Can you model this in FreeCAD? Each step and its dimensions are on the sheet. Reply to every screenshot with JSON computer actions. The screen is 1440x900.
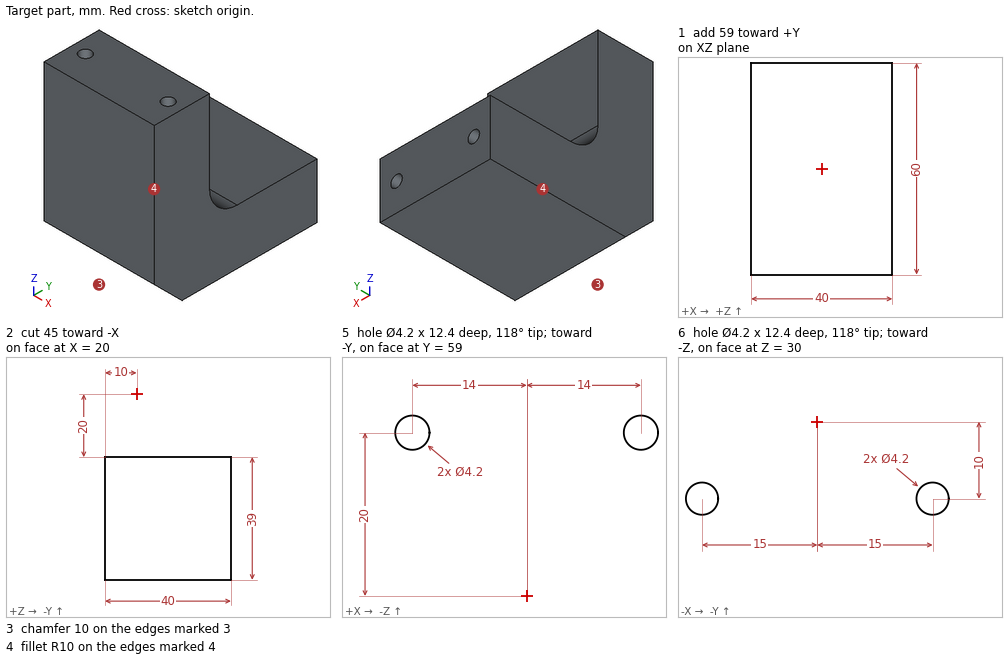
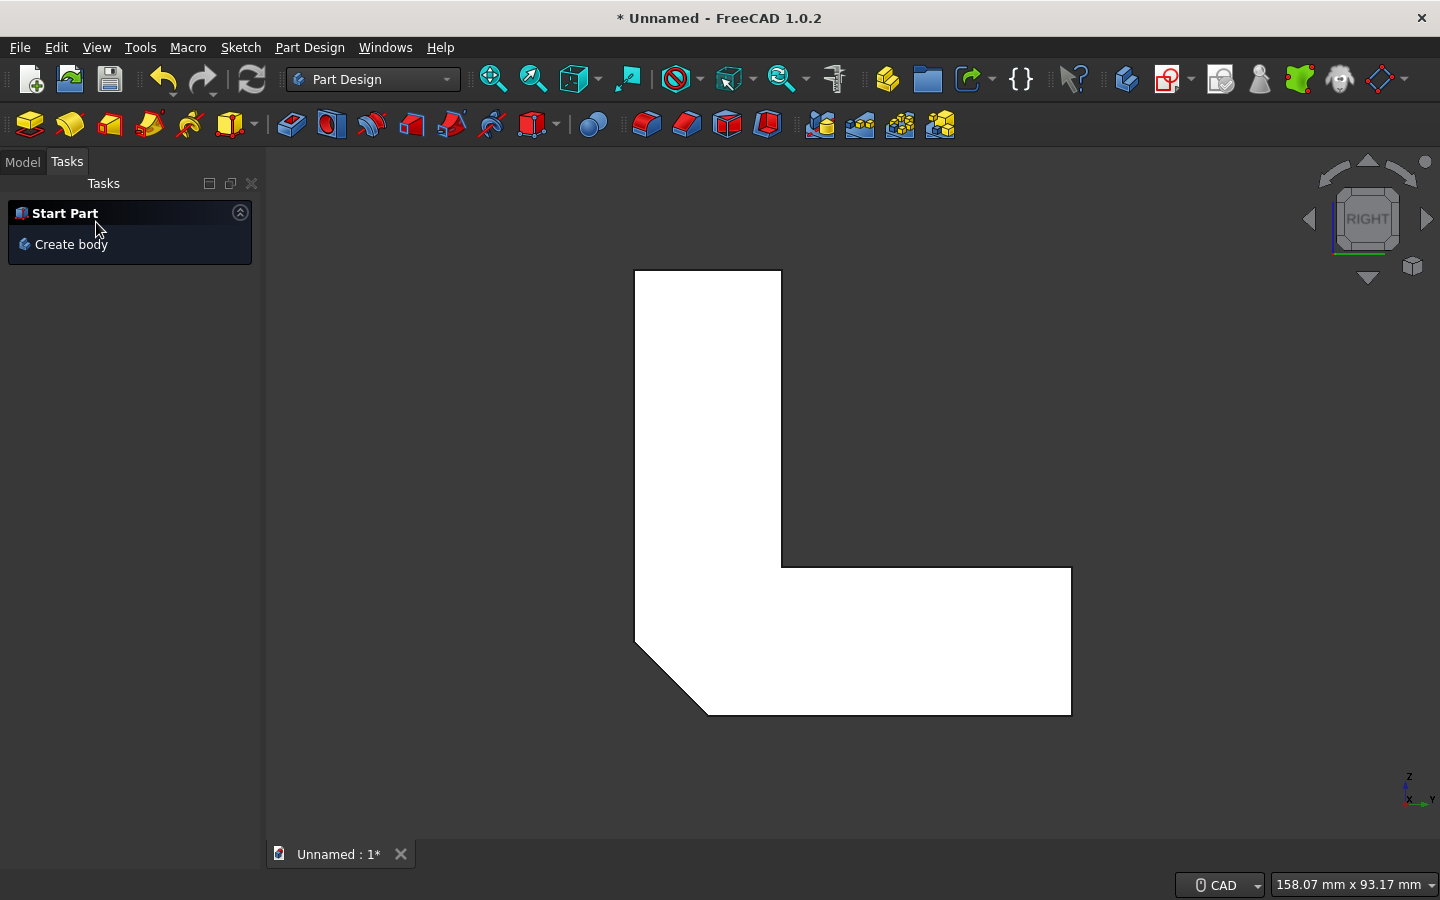
{"action": "key", "text": "5"}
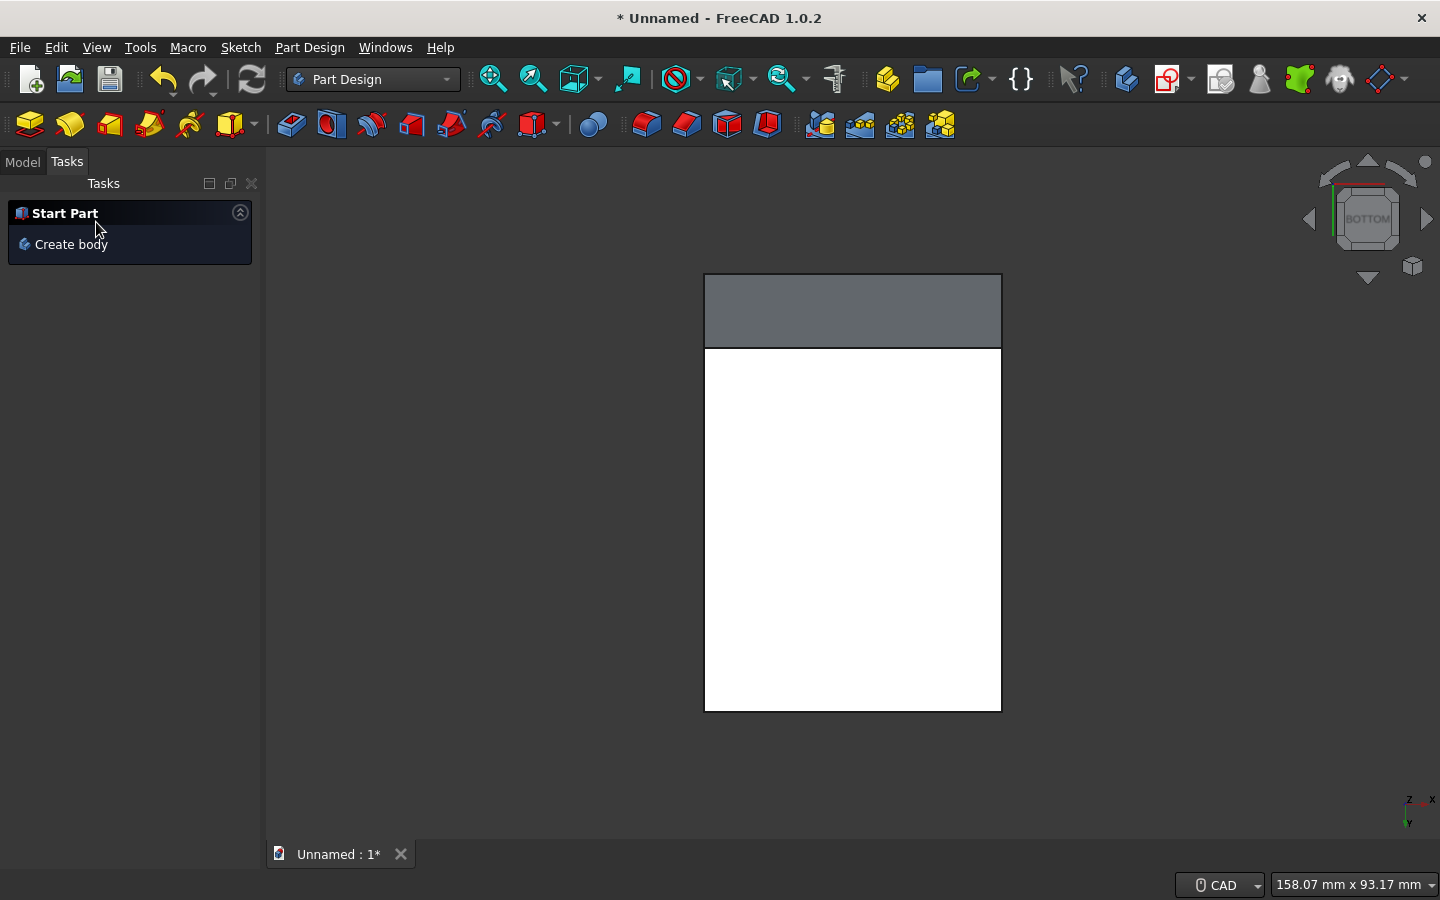
{"action": "key", "text": "4"}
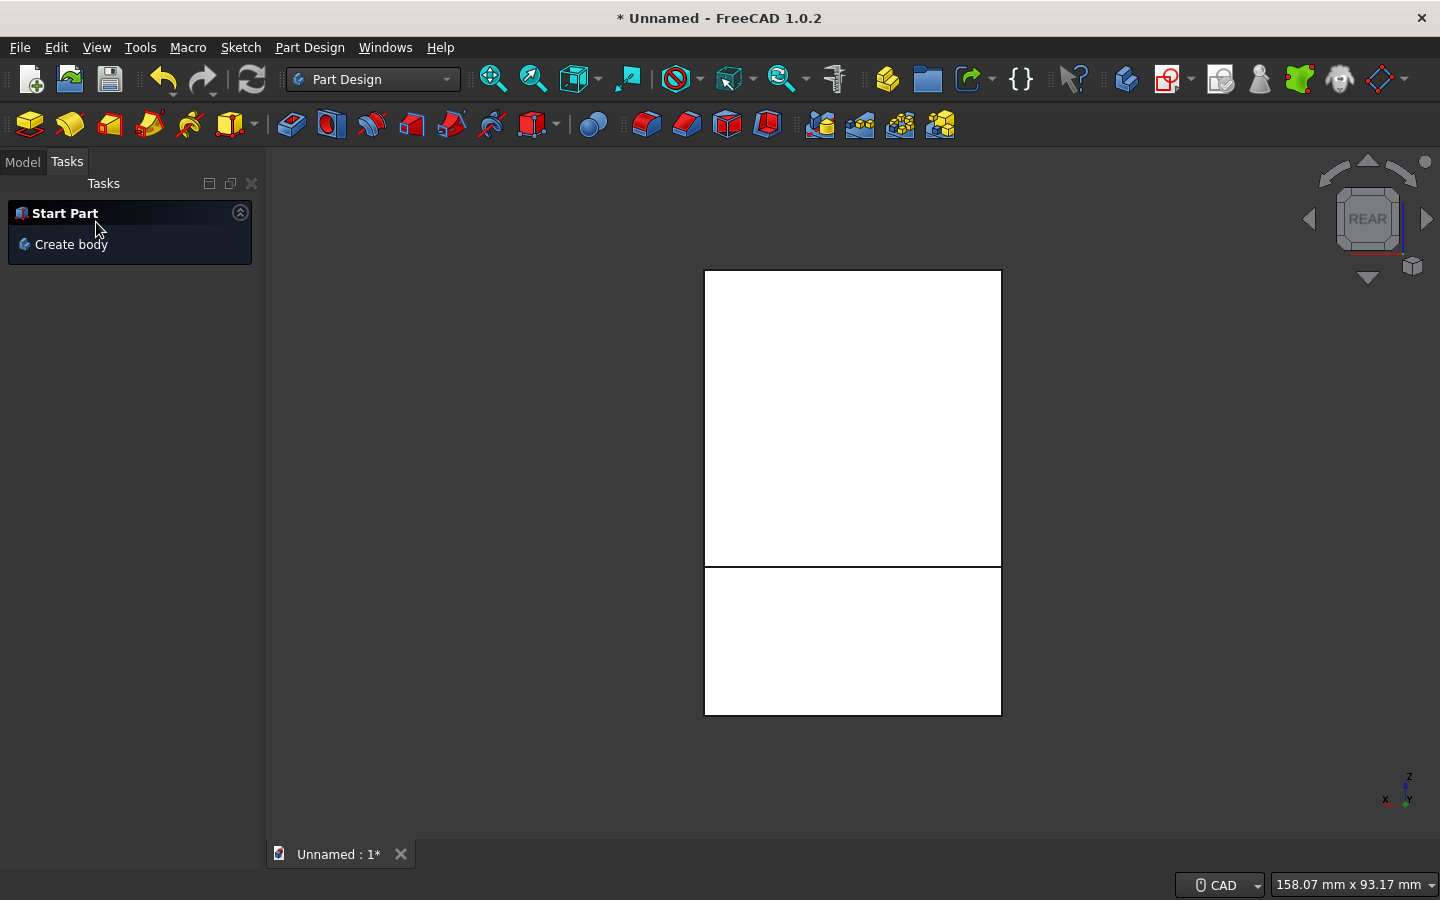
{"action": "key", "text": "6"}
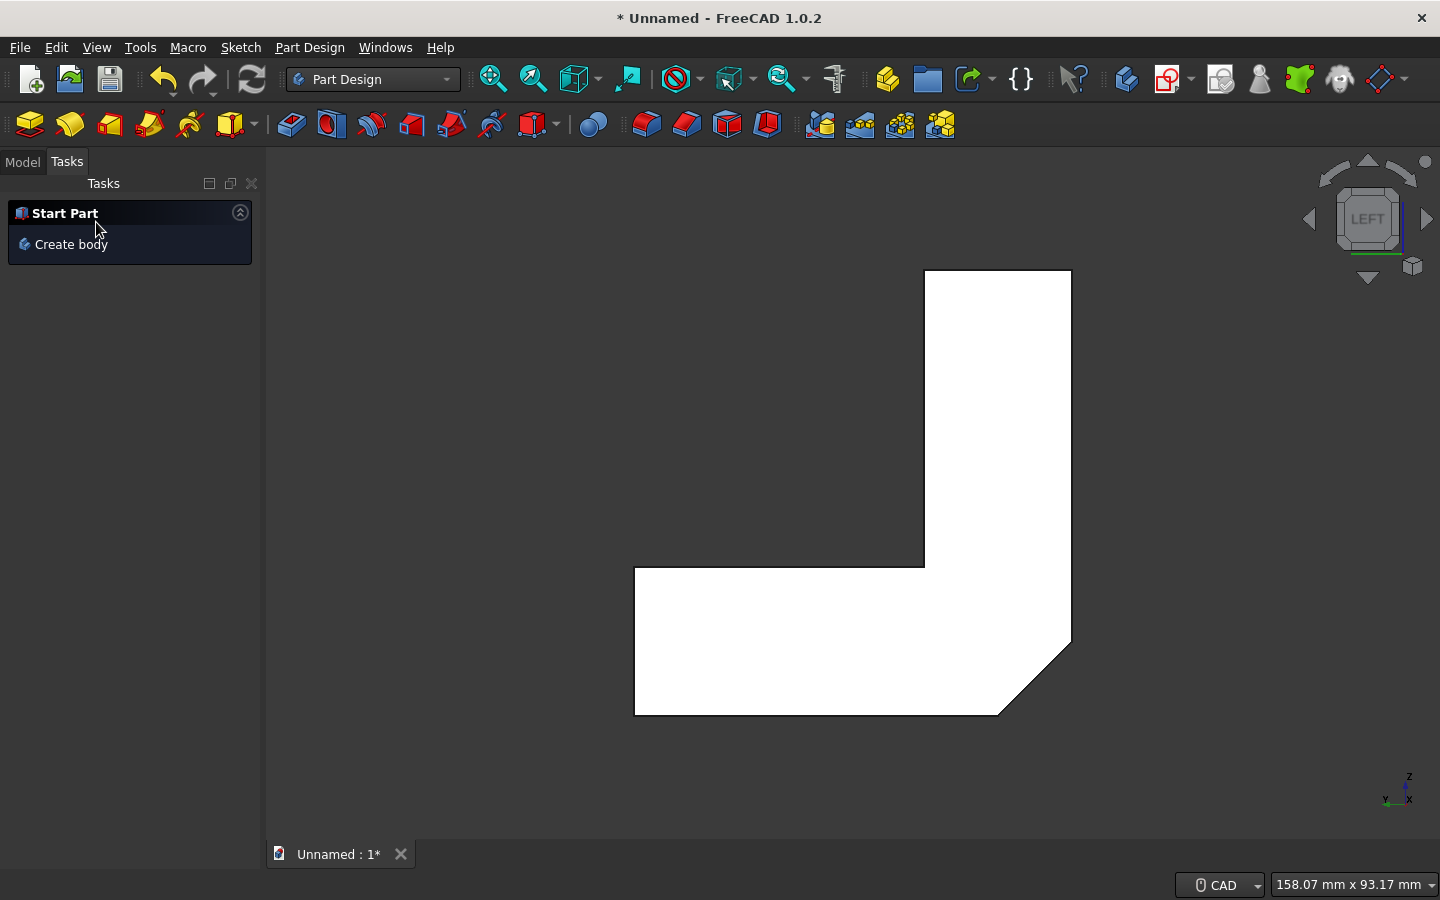
{"action": "key", "text": "v 3"}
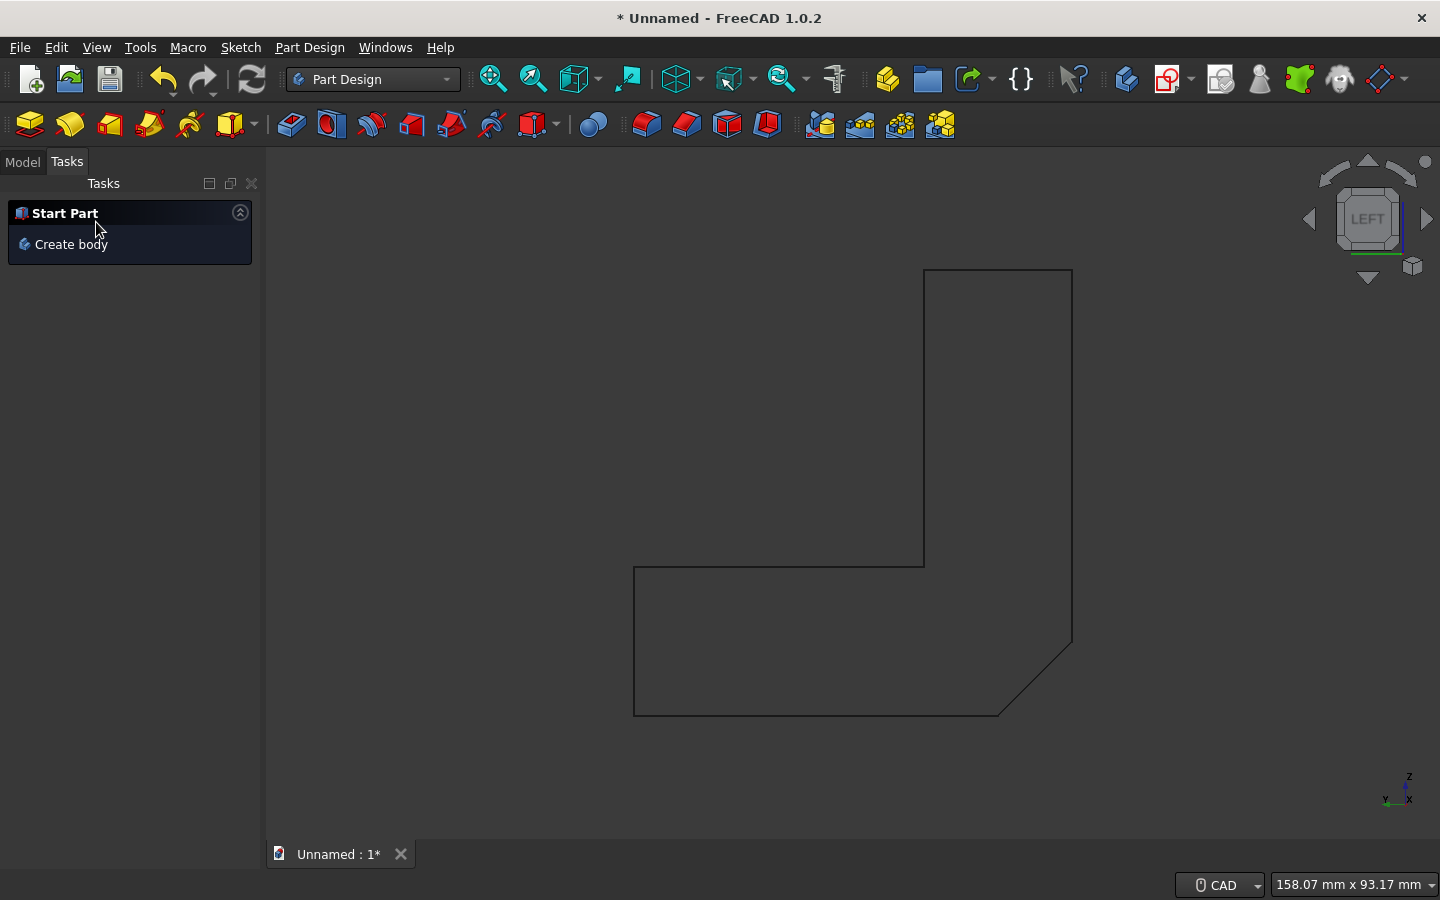
{"action": "key", "text": "0"}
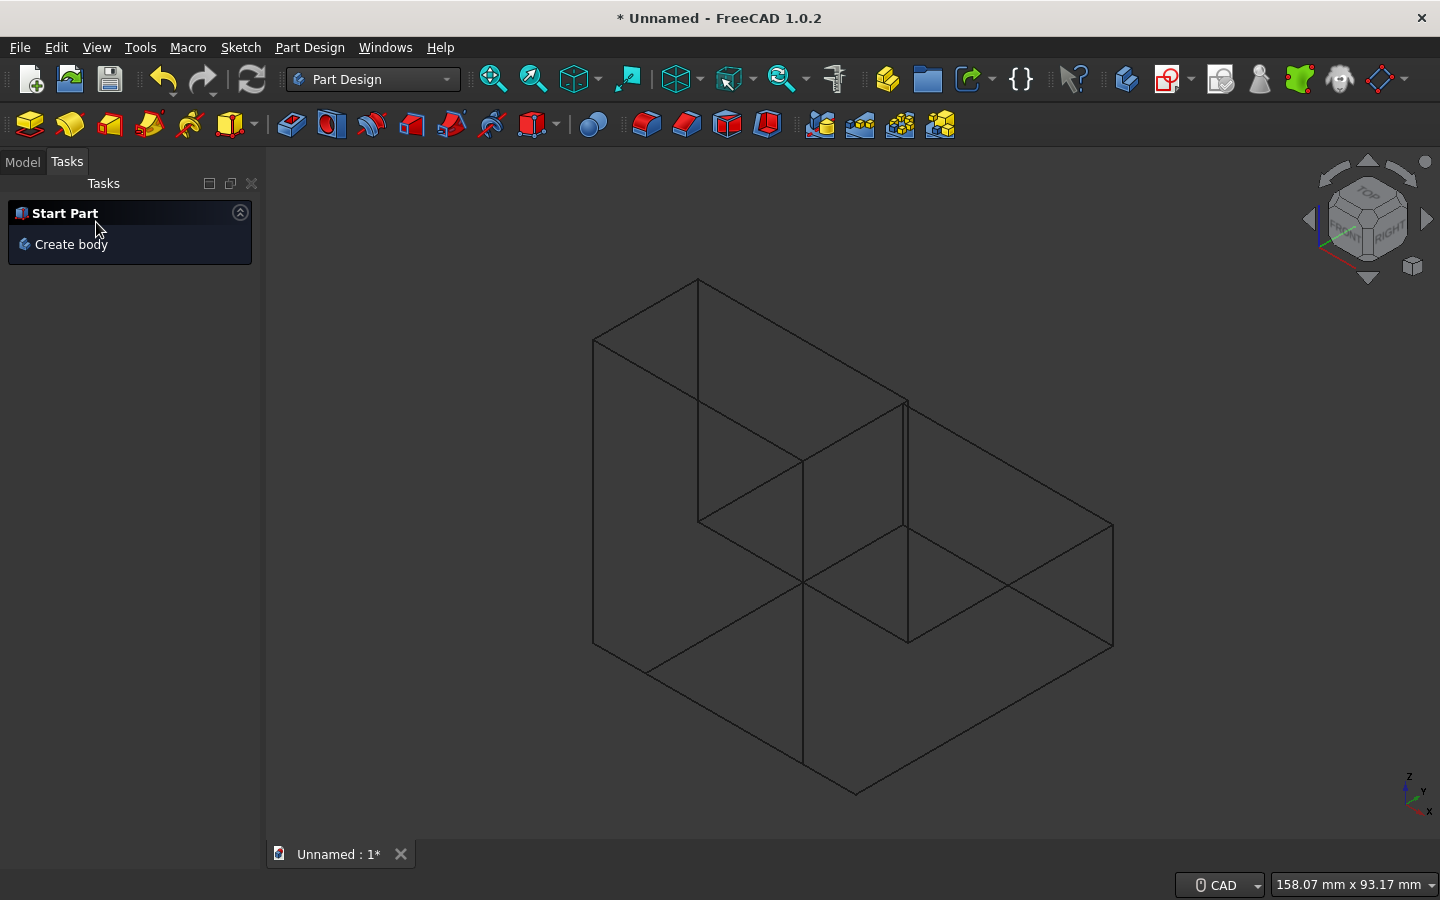
{"action": "left_click", "coordinate": [824, 594]}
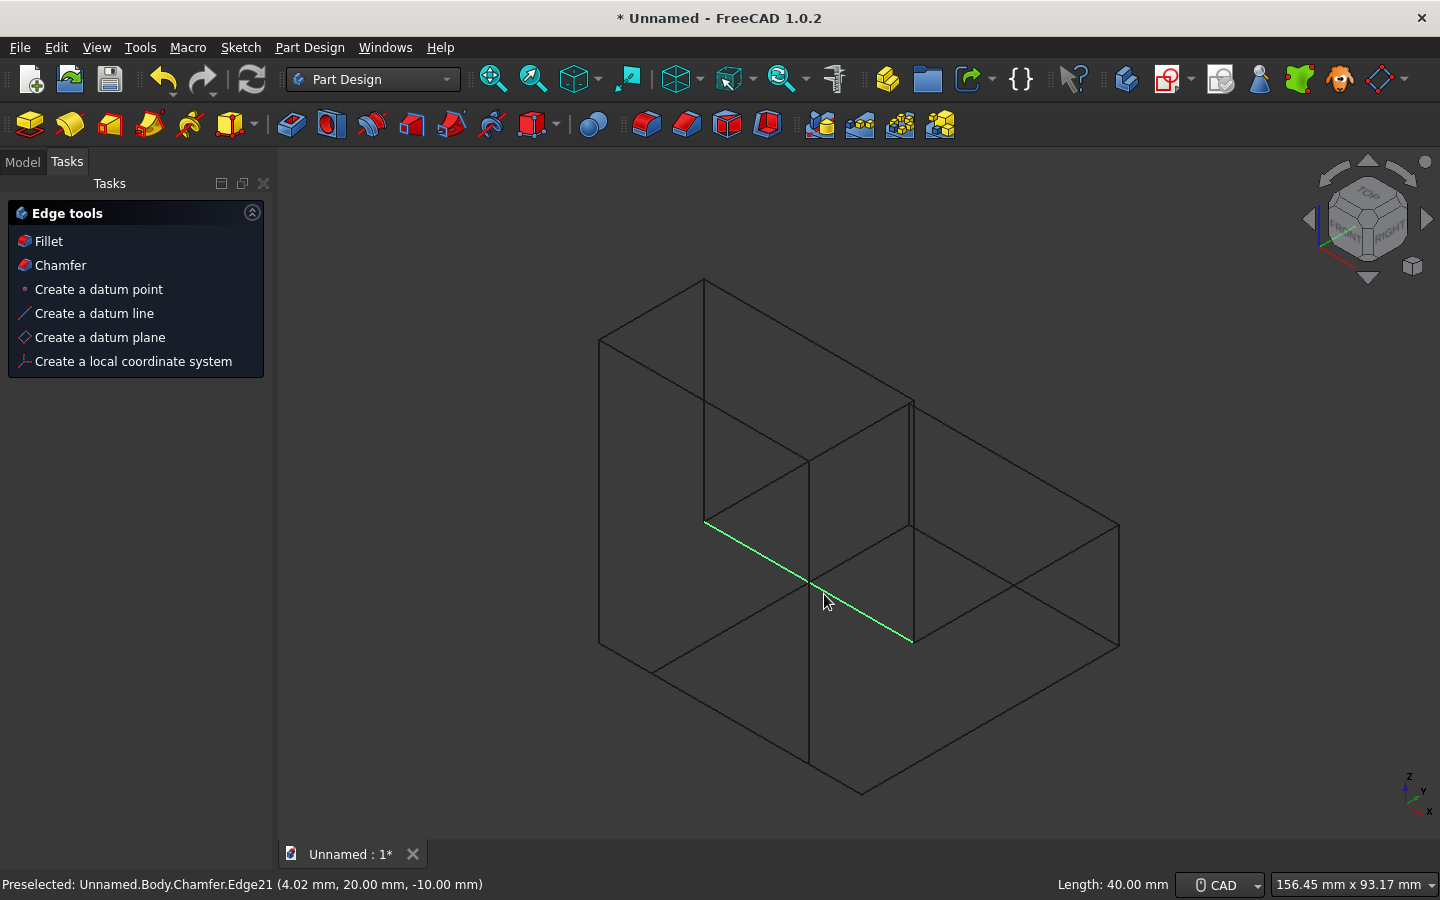
{"action": "key", "text": "v 1"}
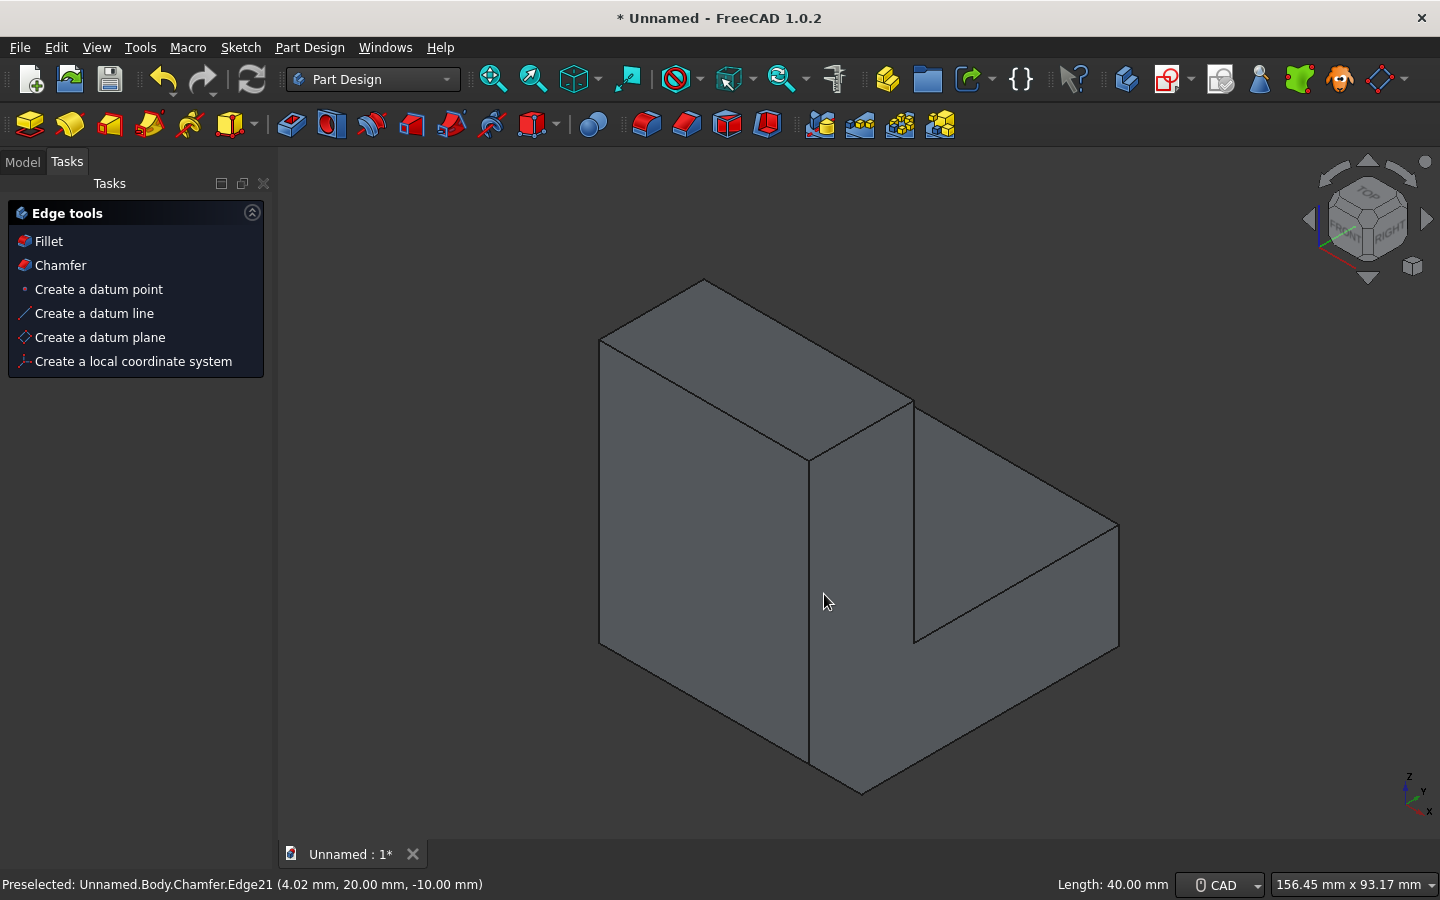
{"action": "left_click", "coordinate": [648, 124]}